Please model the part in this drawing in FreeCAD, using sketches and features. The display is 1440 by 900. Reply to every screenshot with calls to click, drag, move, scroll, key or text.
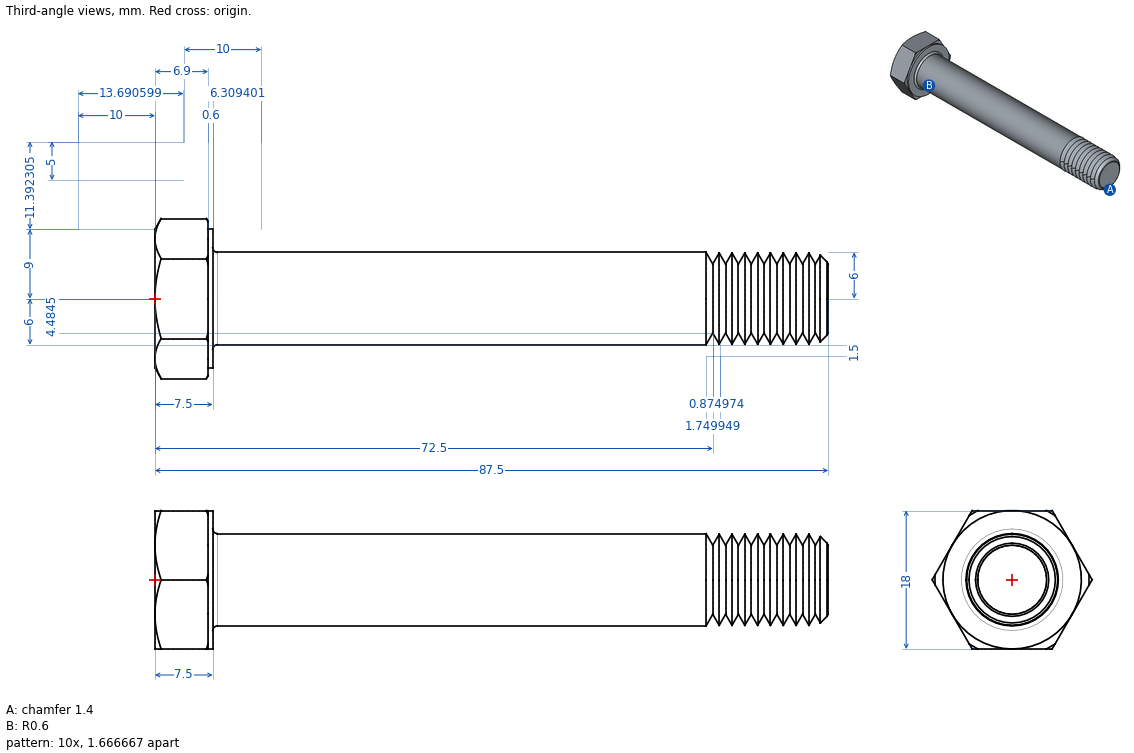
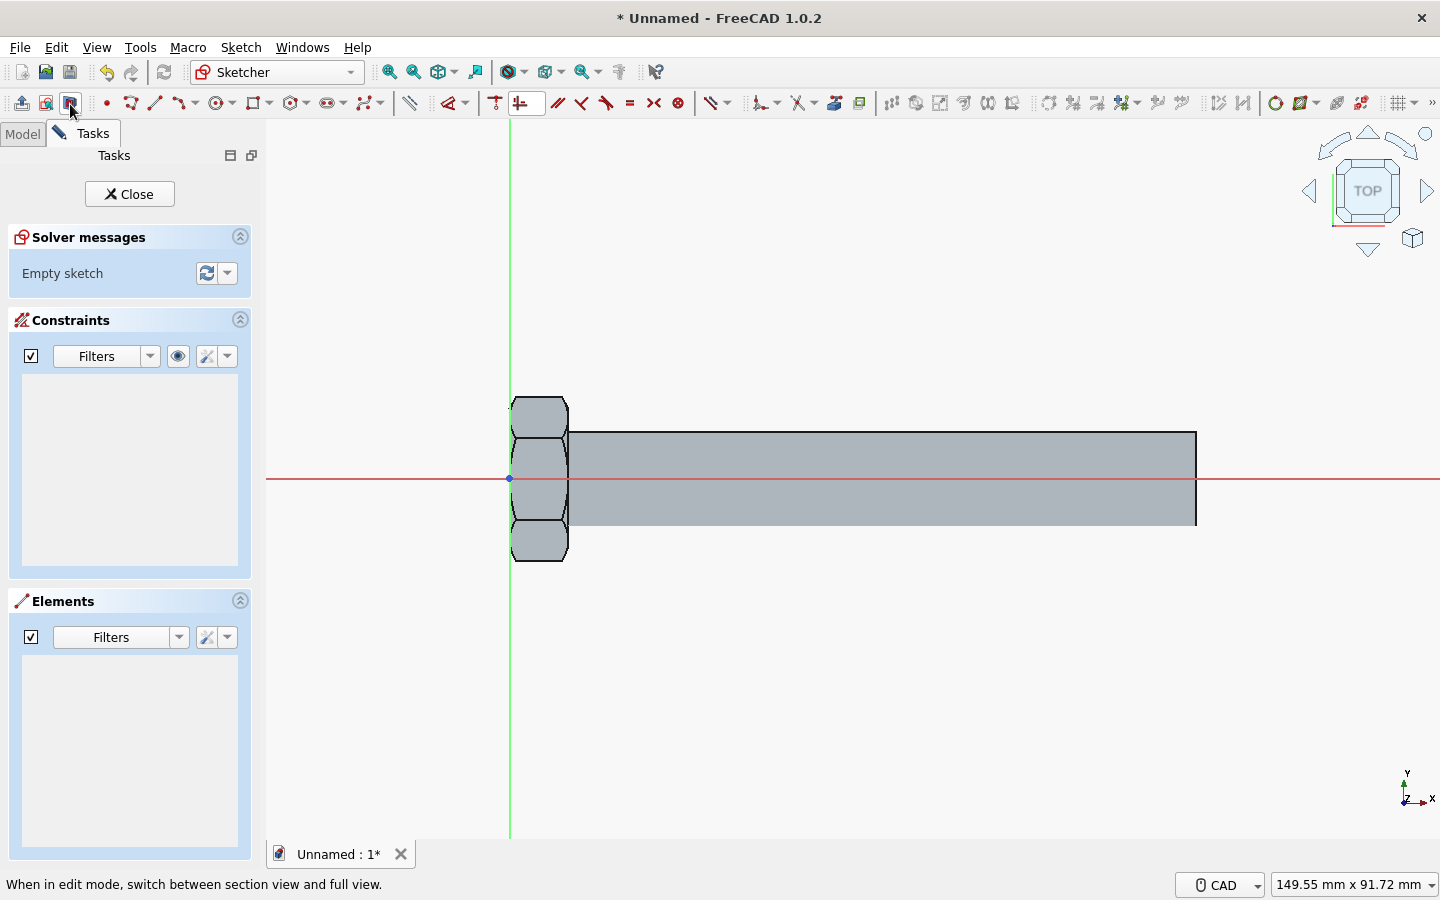
scroll(396, 352, up, 5)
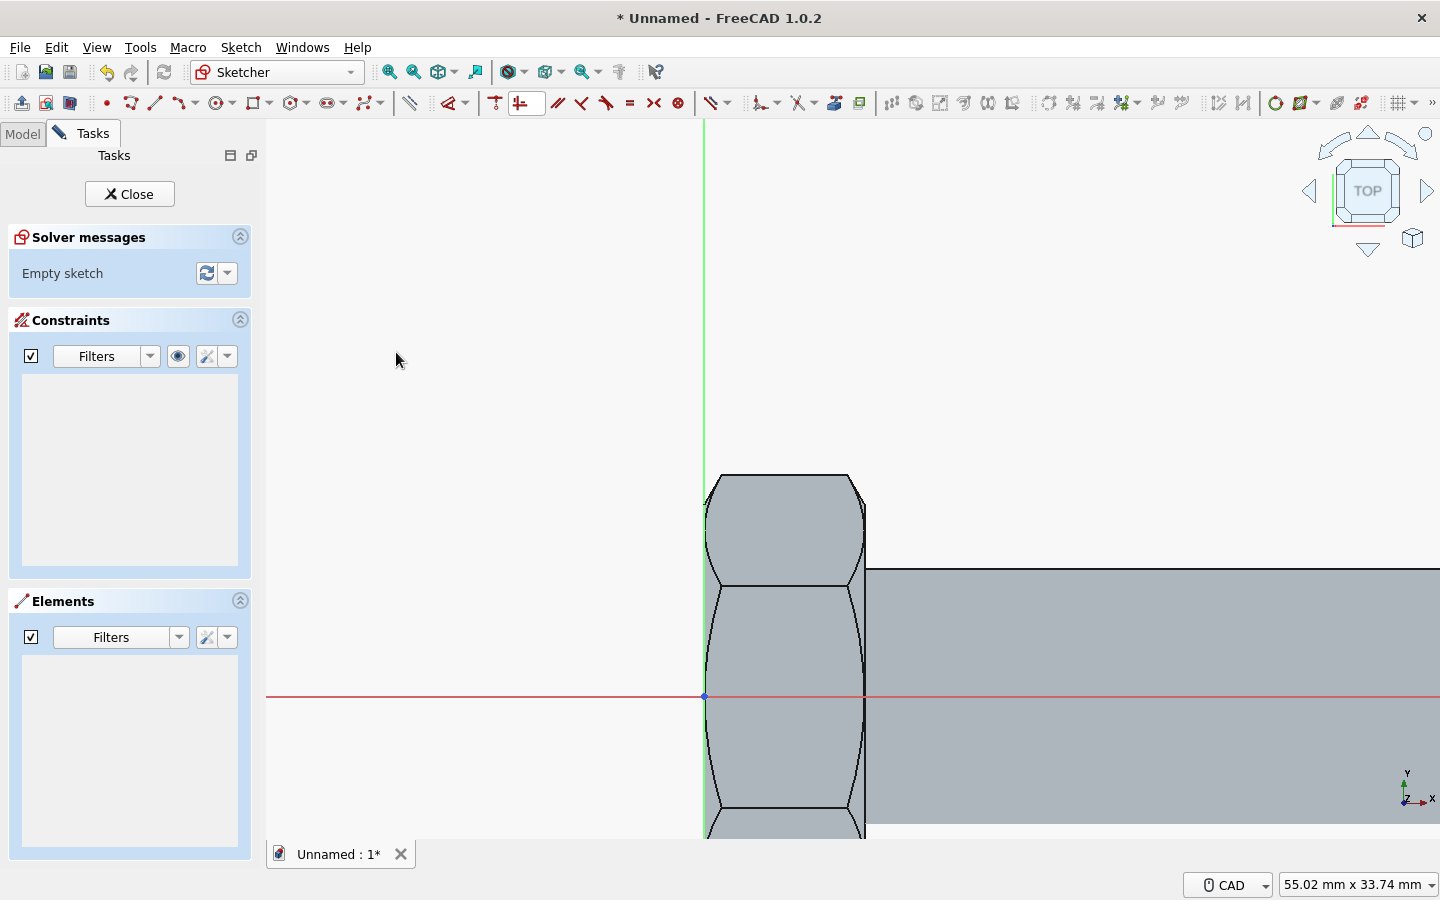
click(254, 104)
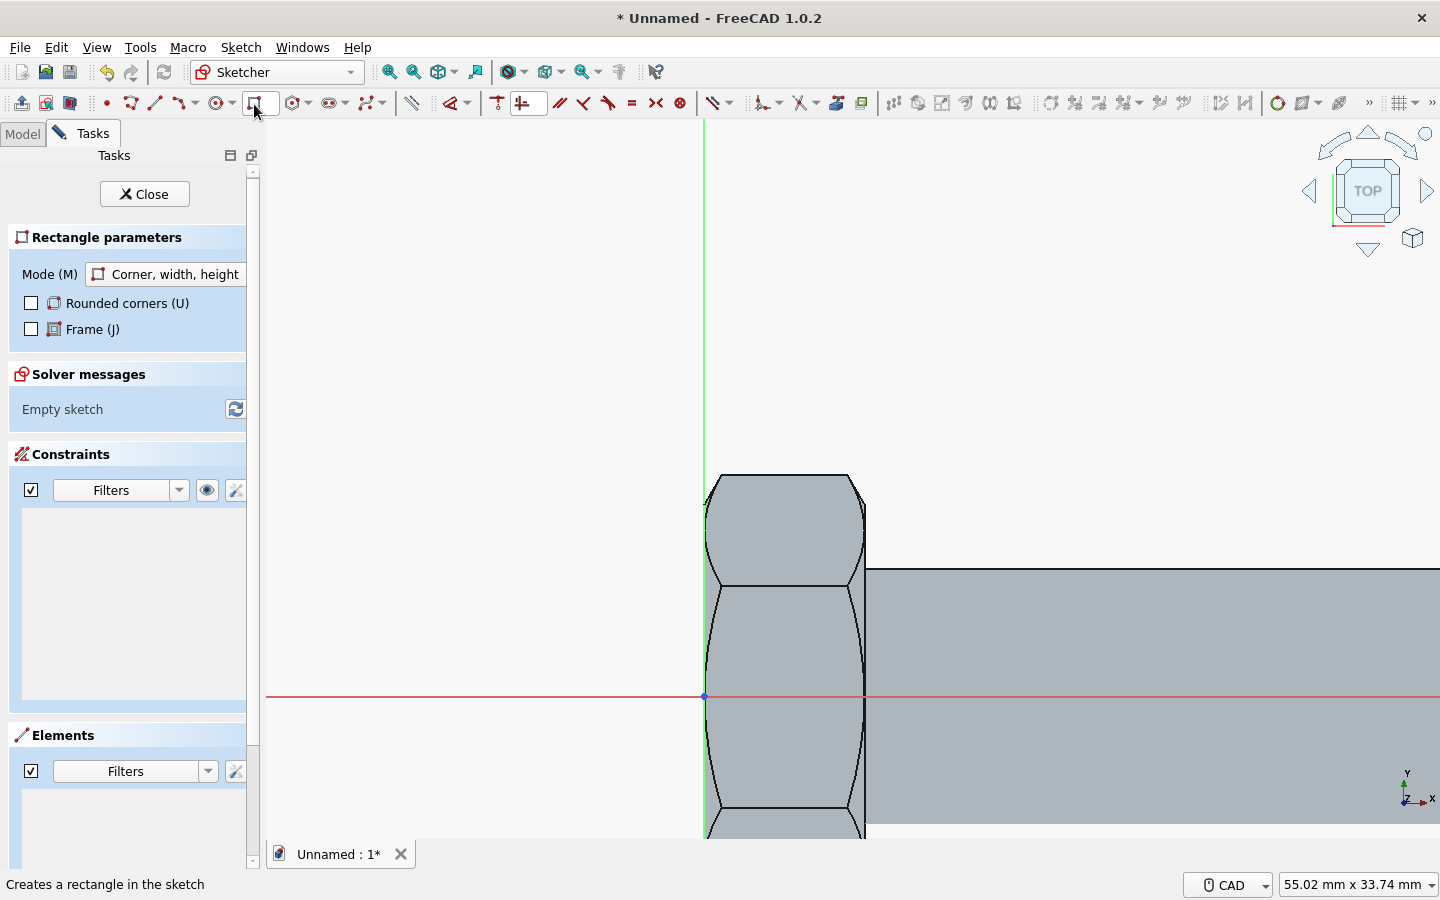
scroll(852, 262, up, 2)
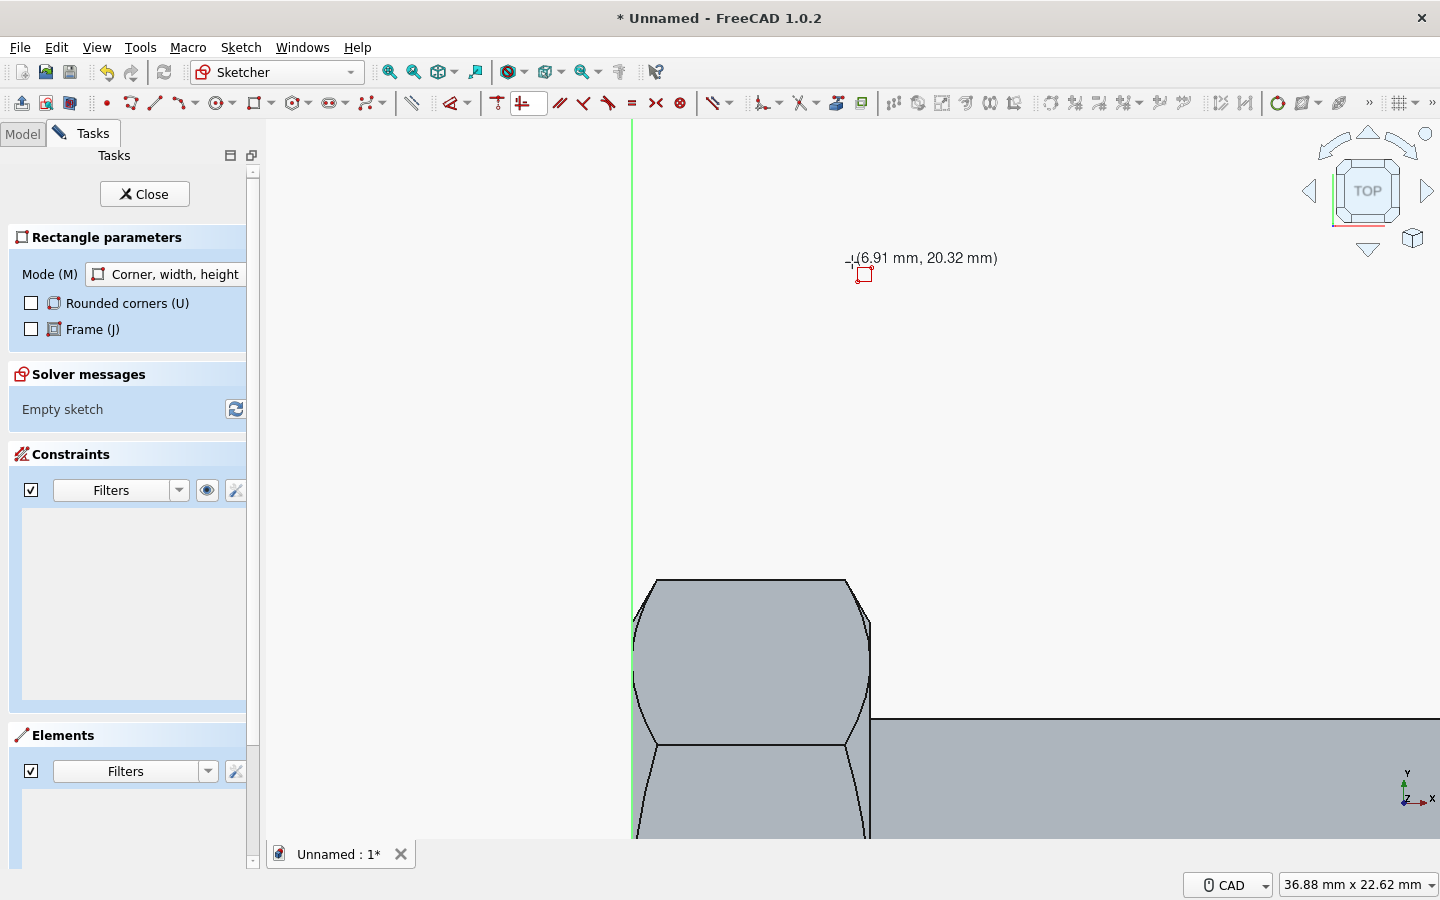
click(851, 261)
click(870, 624)
key(Escape)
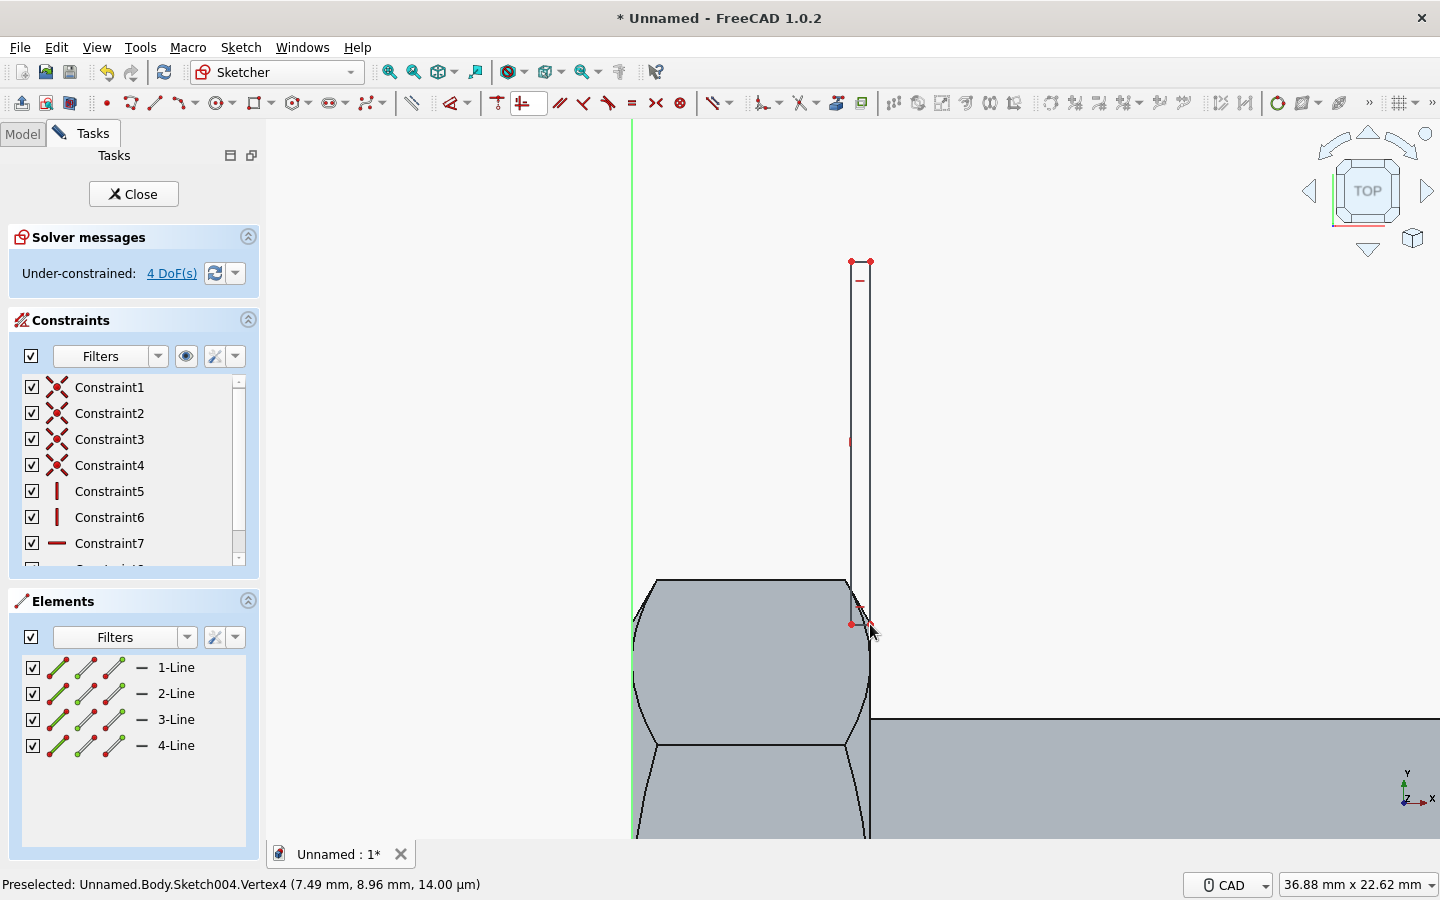
click(450, 104)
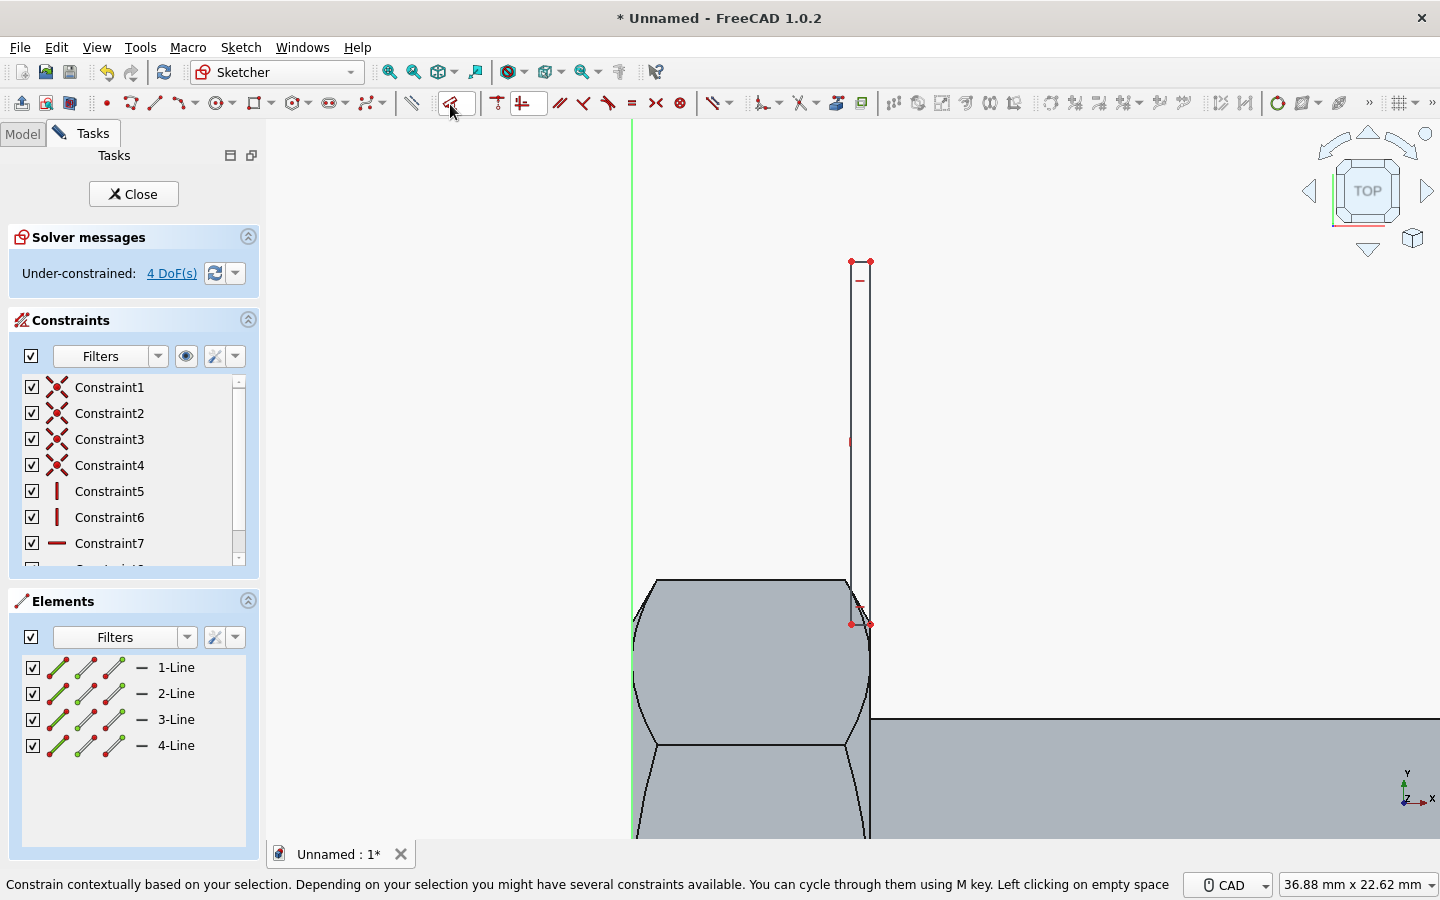
click(851, 625)
click(598, 718)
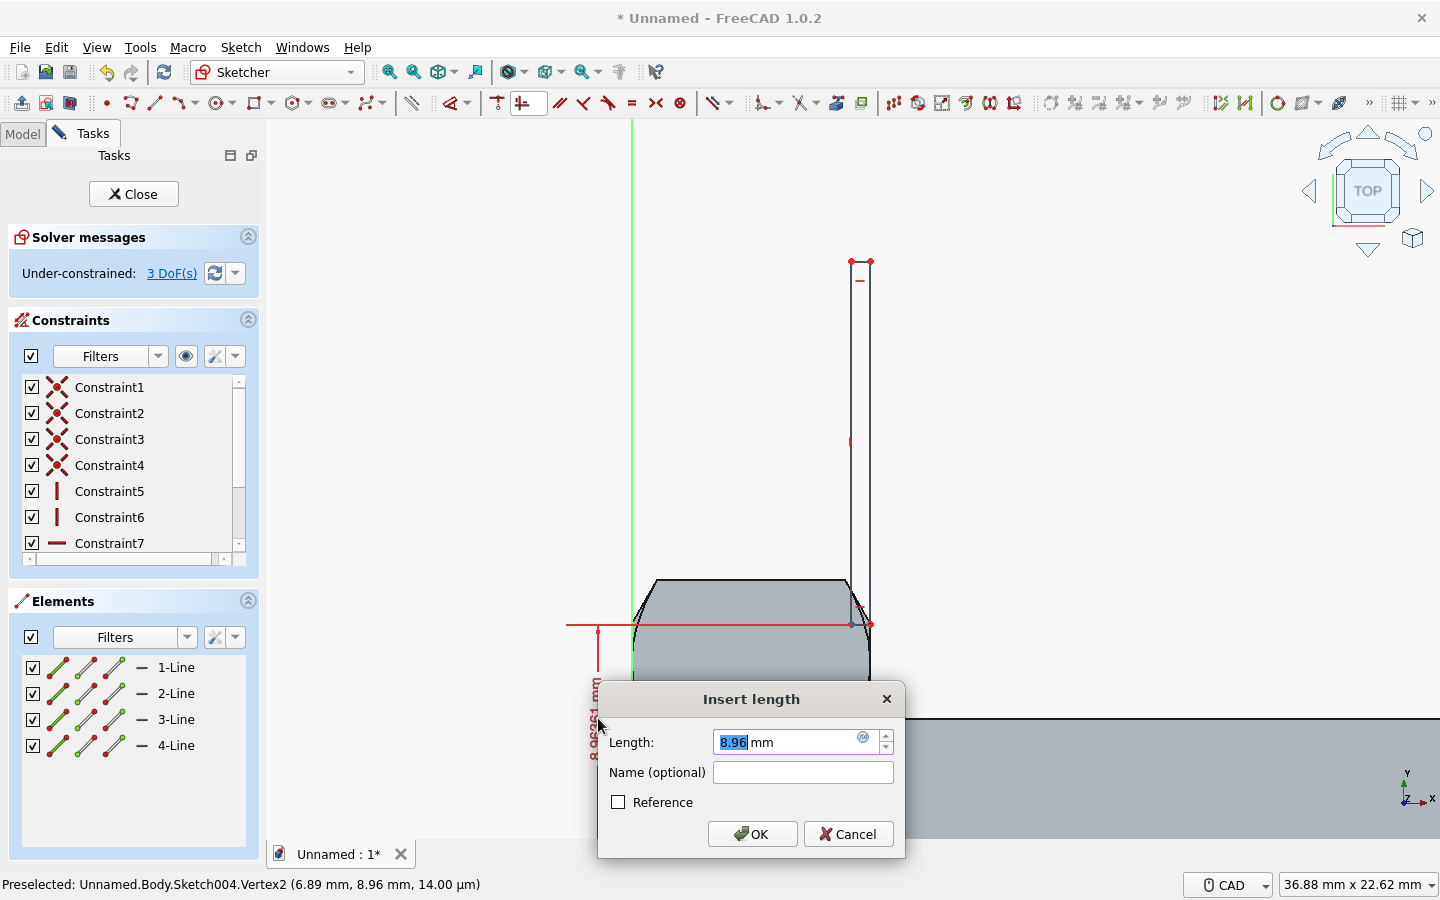
text(9)
key(Return)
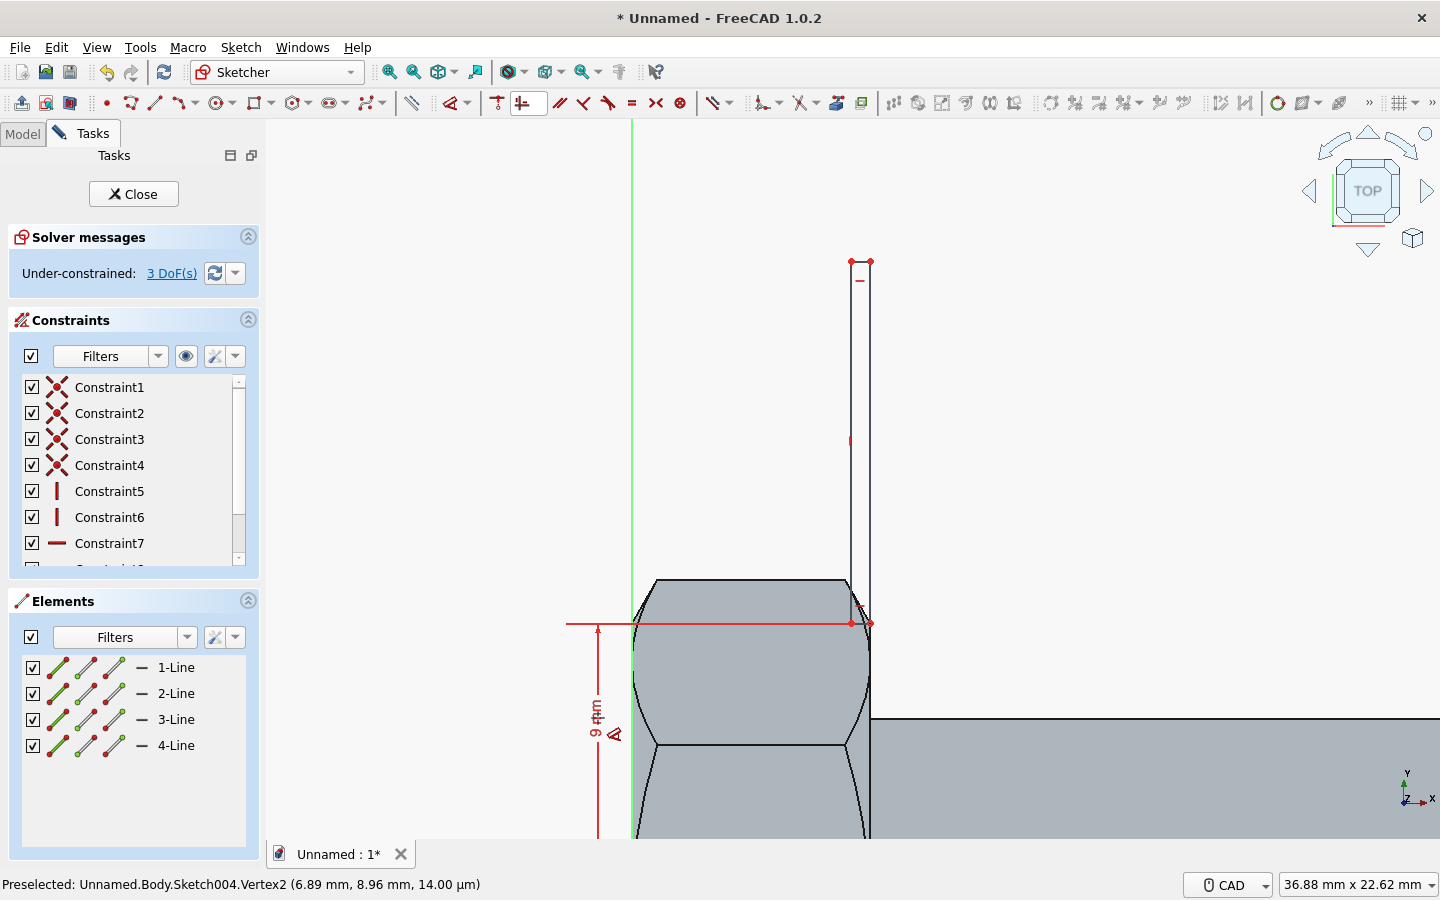
scroll(861, 624, up, 4)